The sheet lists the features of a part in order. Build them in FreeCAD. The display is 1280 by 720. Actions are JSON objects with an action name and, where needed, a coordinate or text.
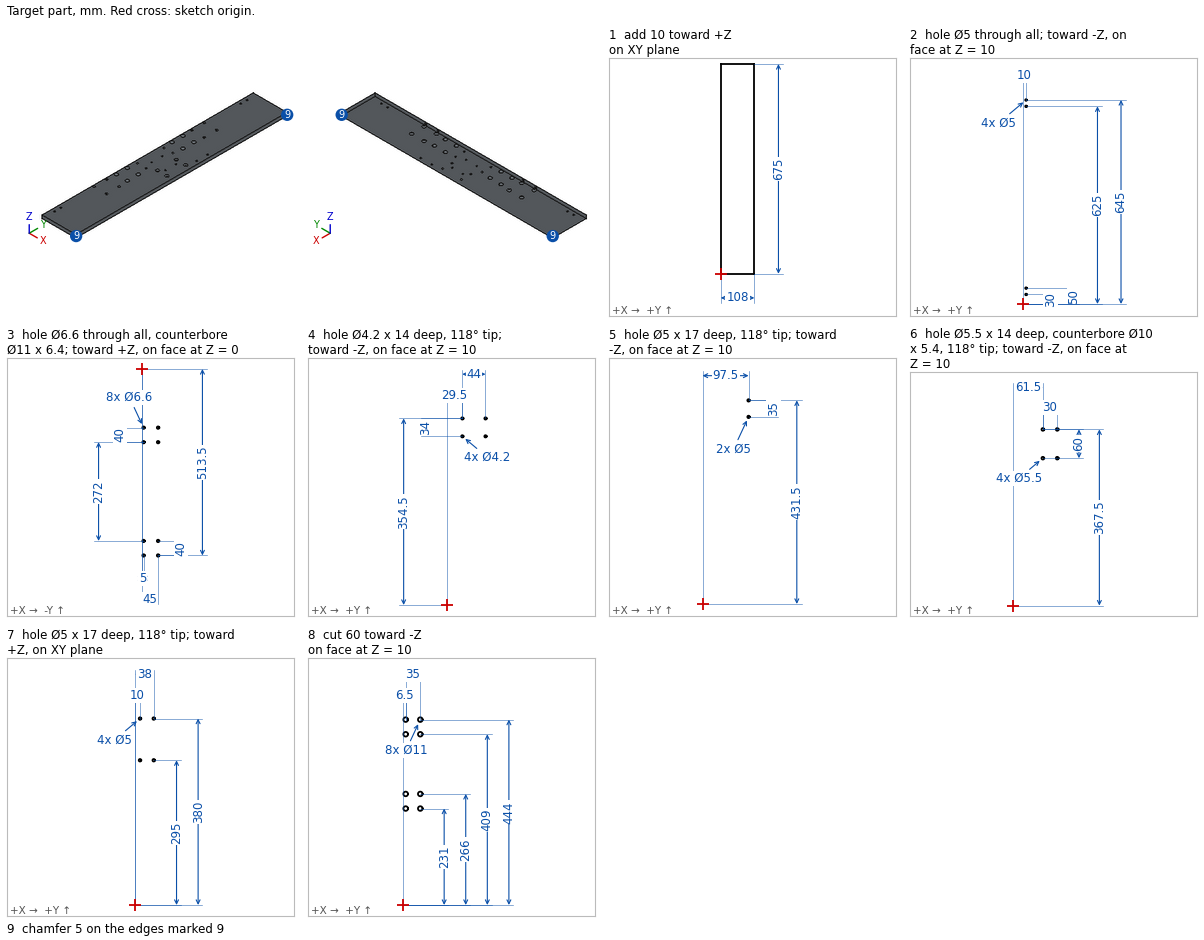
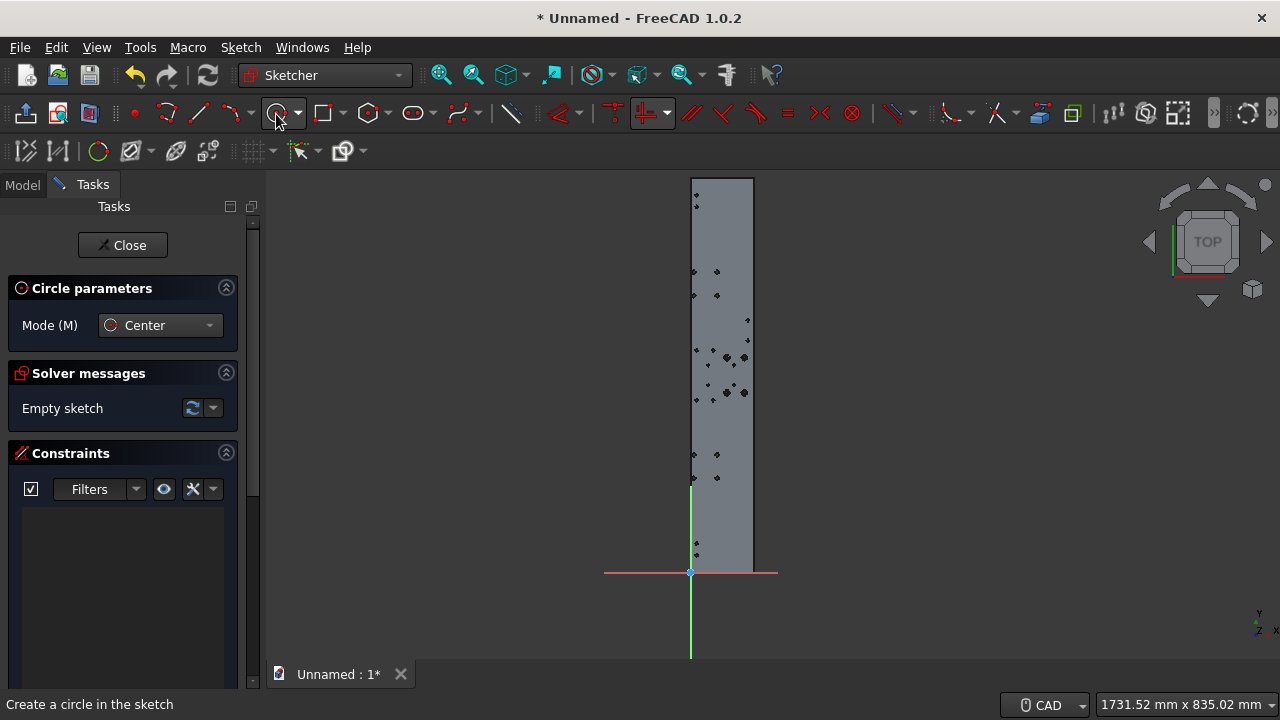
{"action": "scroll", "coordinate": [715, 313], "scroll_direction": "up", "scroll_amount": 10}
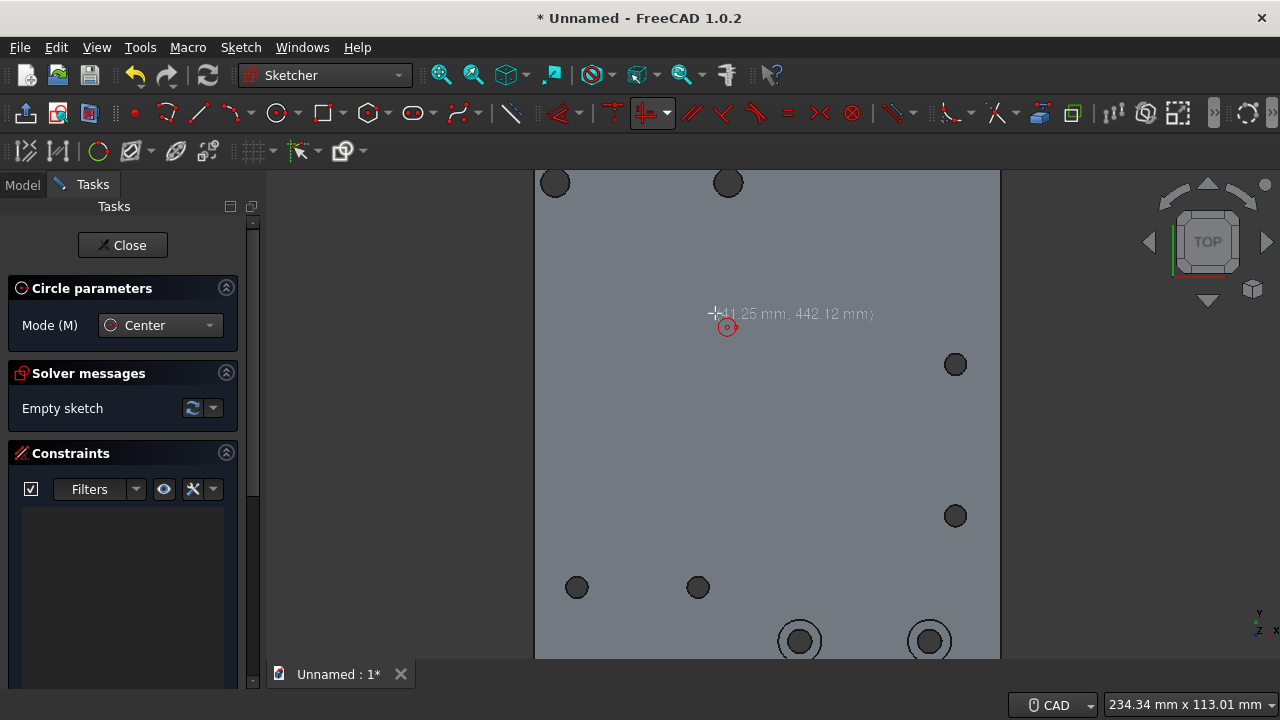
{"action": "scroll", "coordinate": [718, 247], "scroll_direction": "down", "scroll_amount": 9}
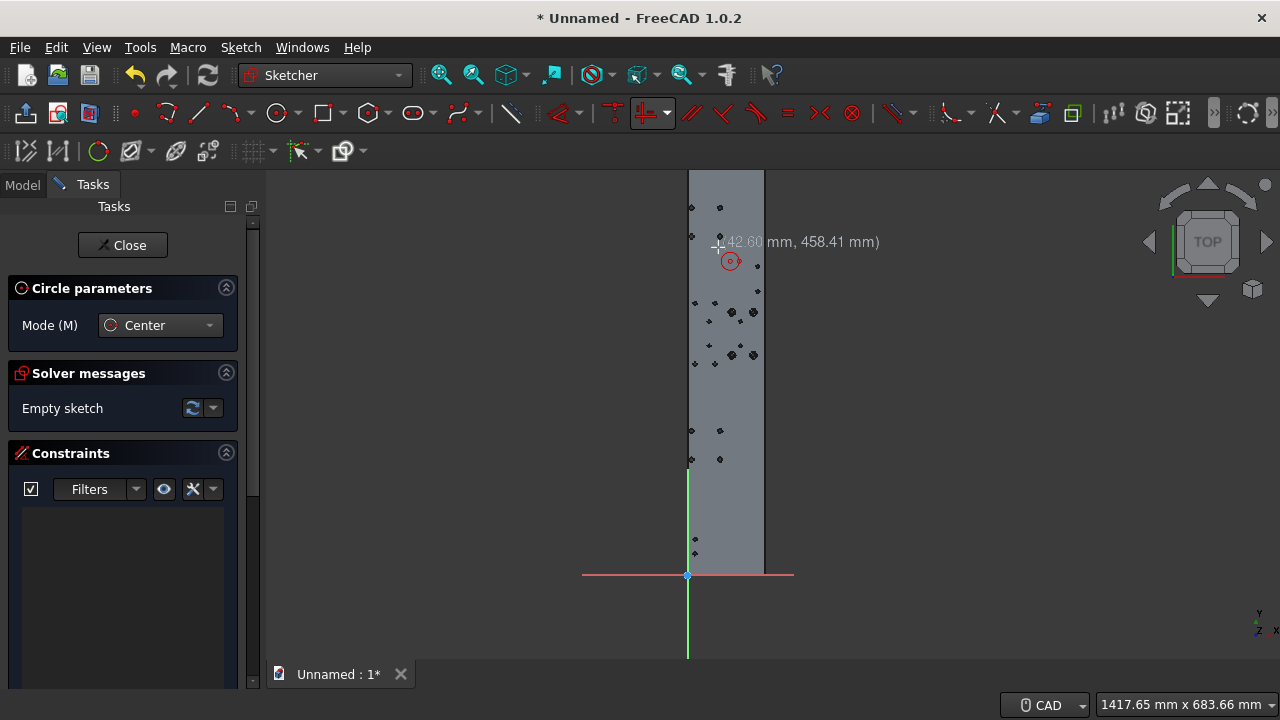
{"action": "left_click", "coordinate": [718, 258]}
{"action": "mouse_move", "coordinate": [720, 255]}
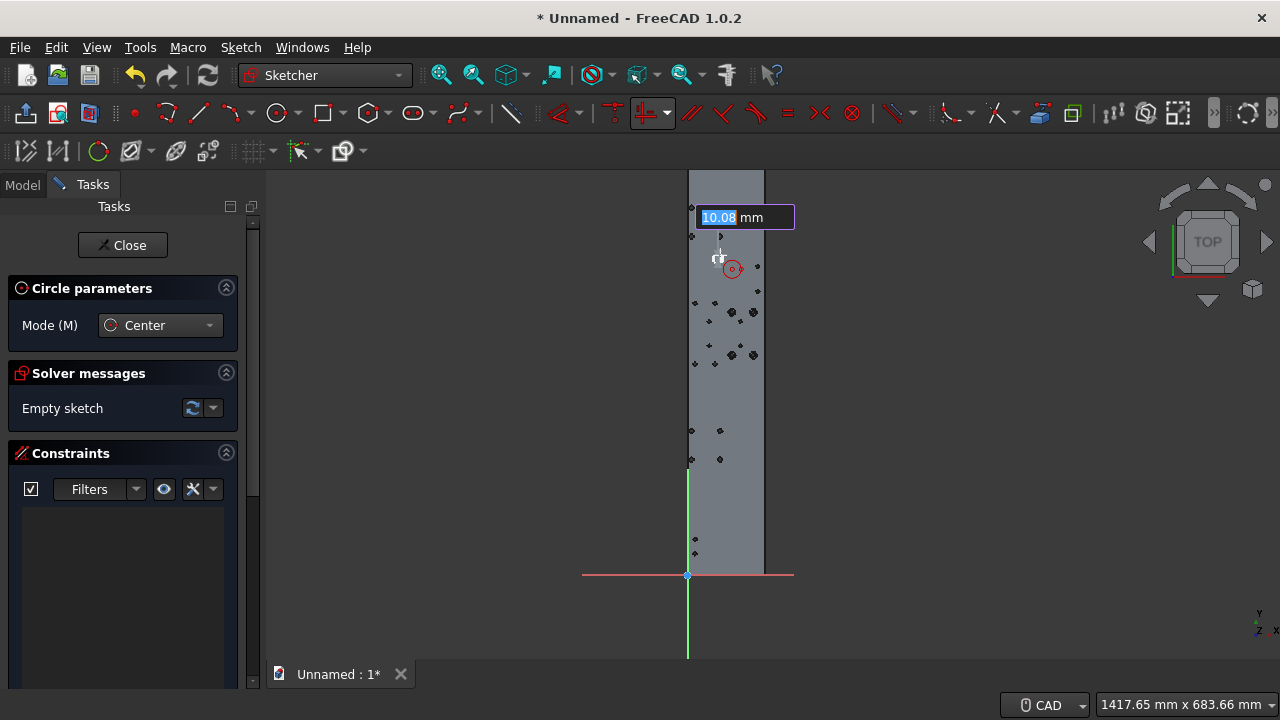
{"action": "type", "text": "11"}
{"action": "key", "text": "Return"}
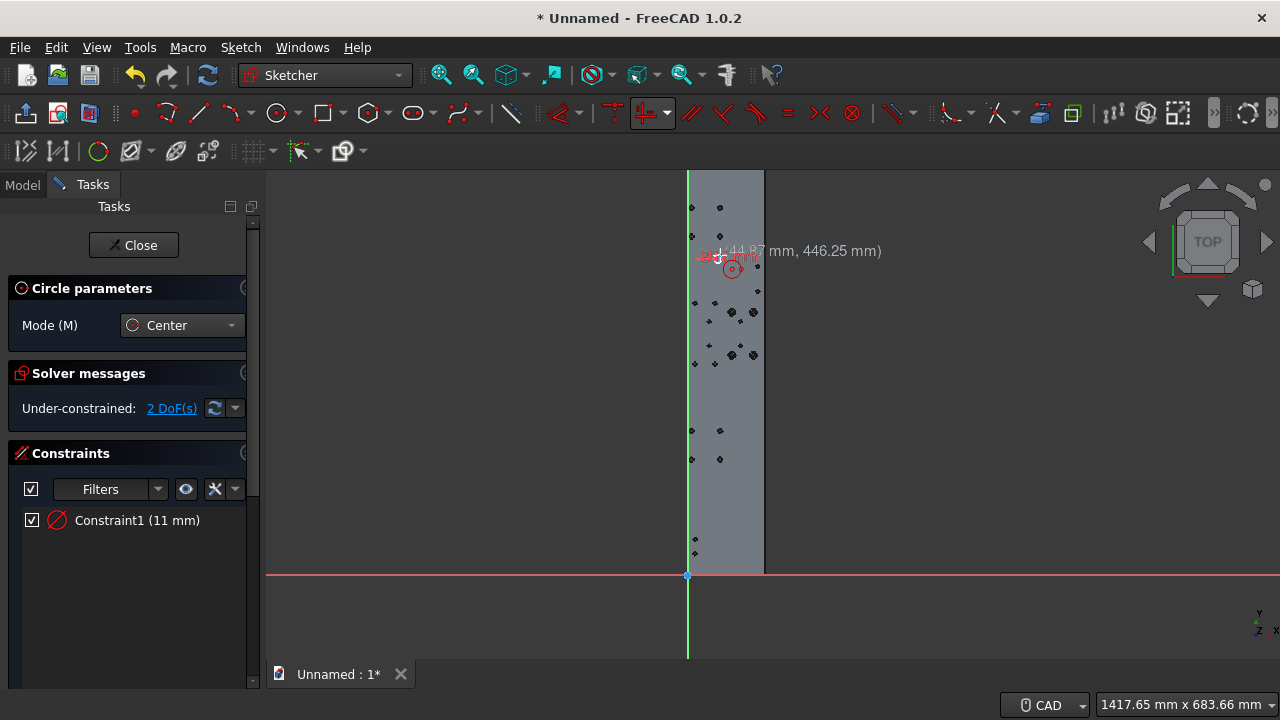
{"action": "scroll", "coordinate": [693, 258], "scroll_direction": "up", "scroll_amount": 9}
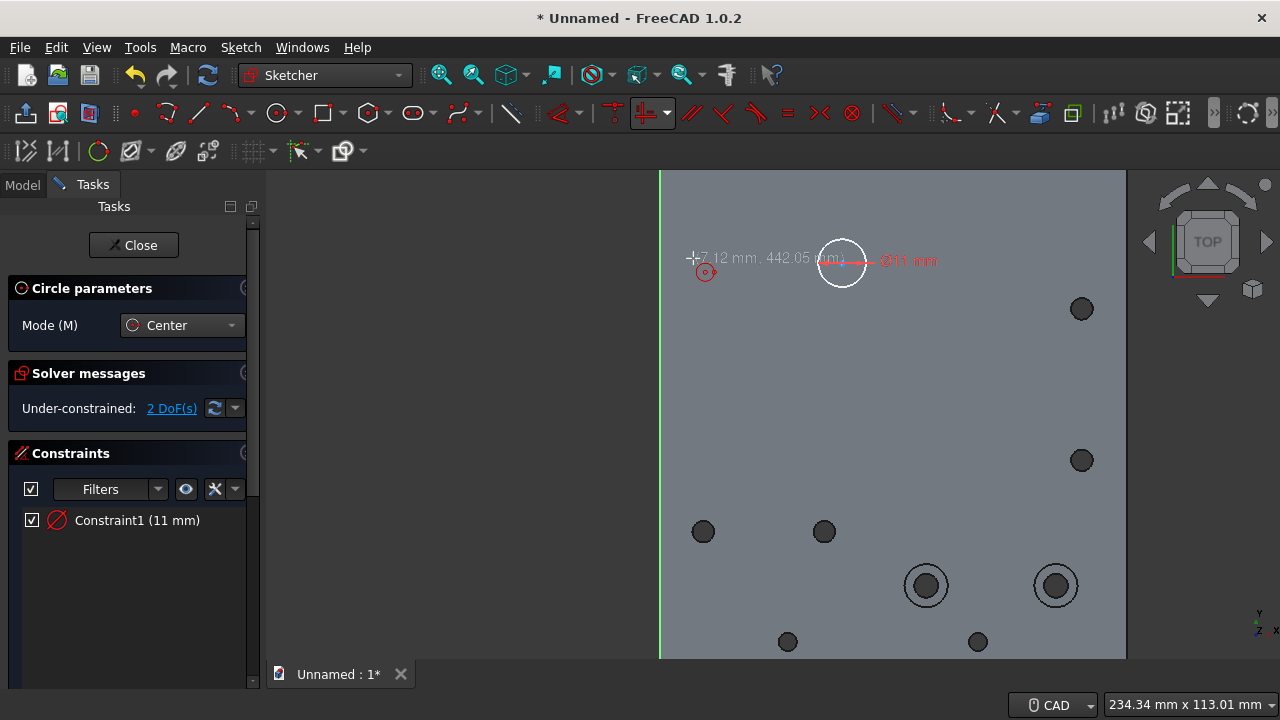
{"action": "left_click", "coordinate": [688, 255]}
{"action": "mouse_move", "coordinate": [705, 238]}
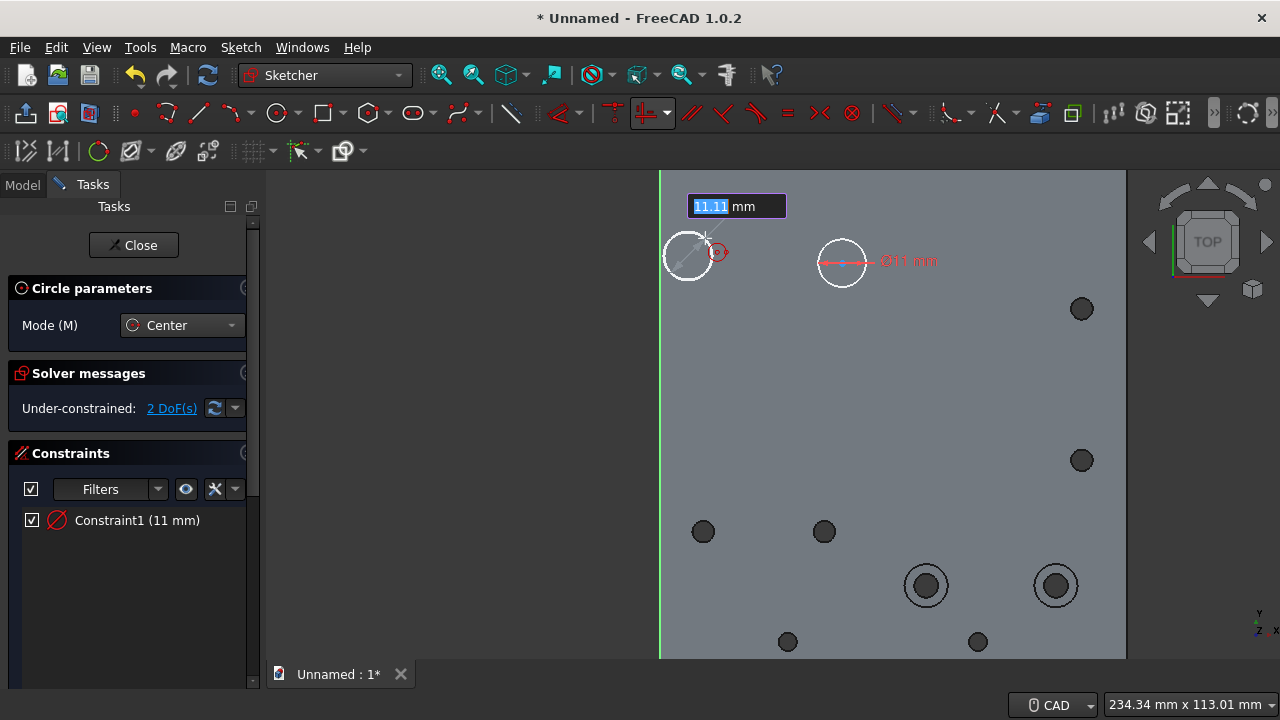
{"action": "type", "text": "11"}
{"action": "key", "text": "Return"}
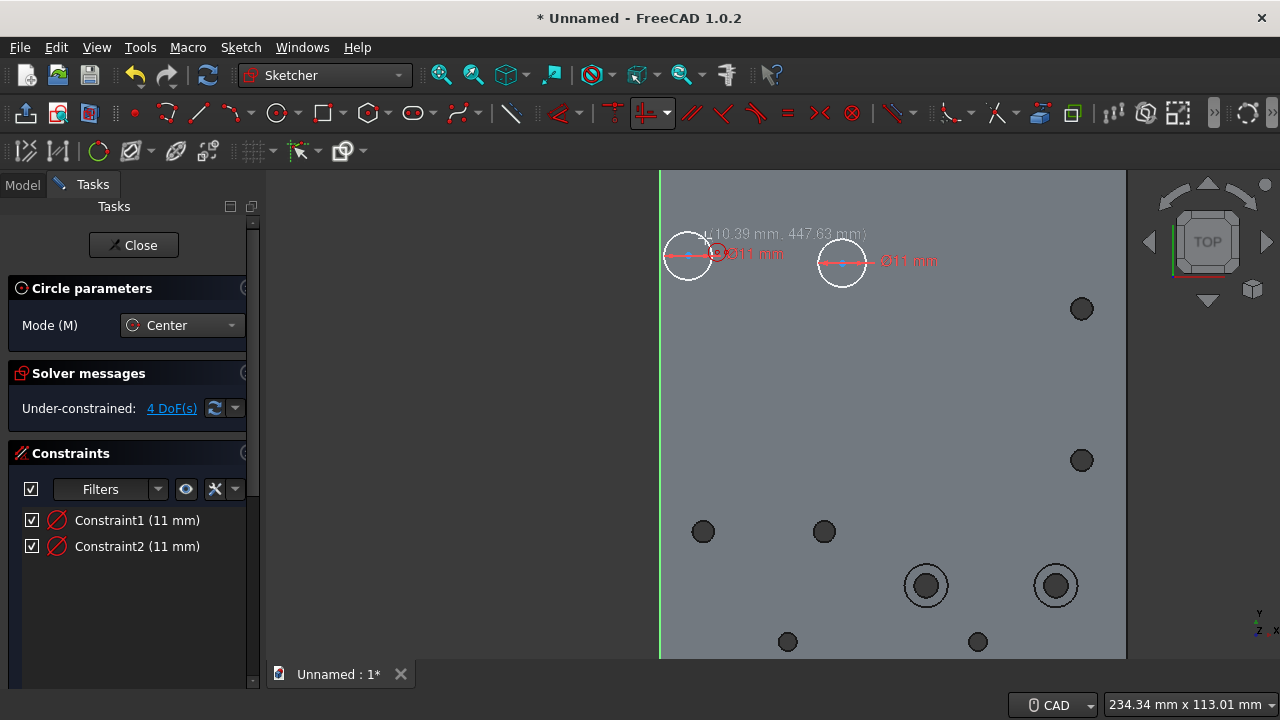
{"action": "scroll", "coordinate": [693, 258], "scroll_direction": "down", "scroll_amount": 9}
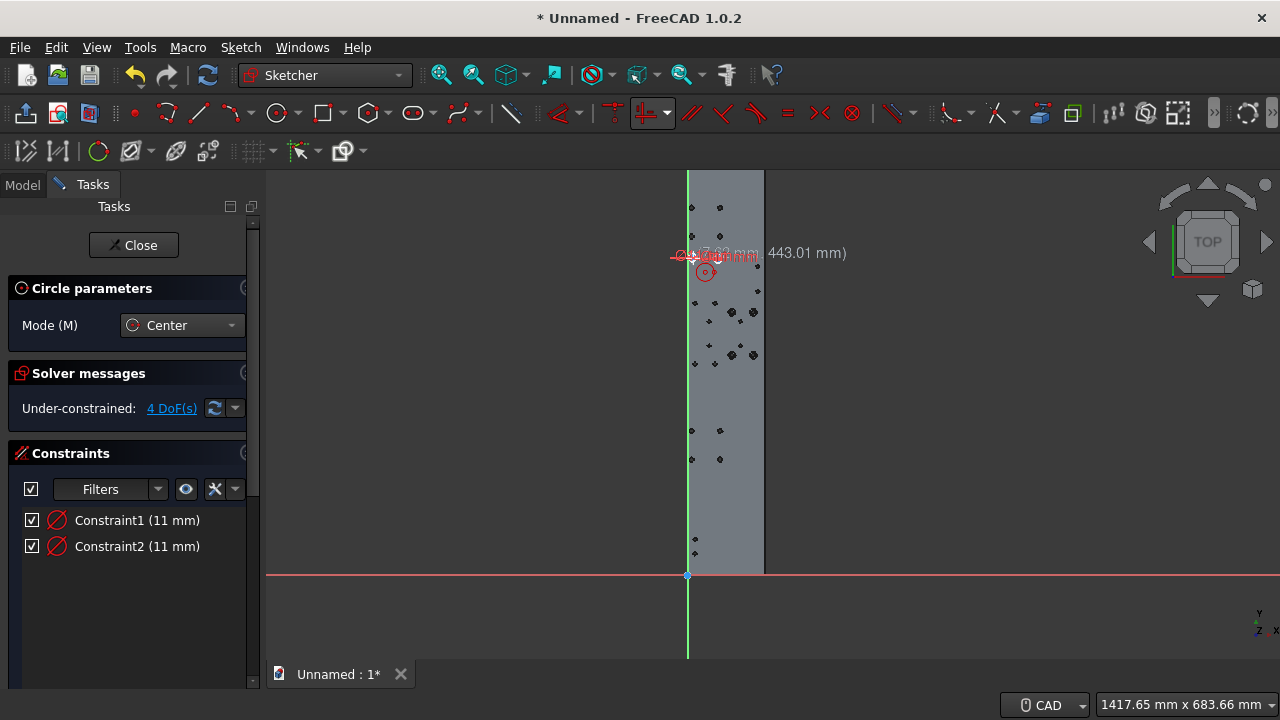
{"action": "left_click", "coordinate": [718, 283]}
{"action": "mouse_move", "coordinate": [720, 280]}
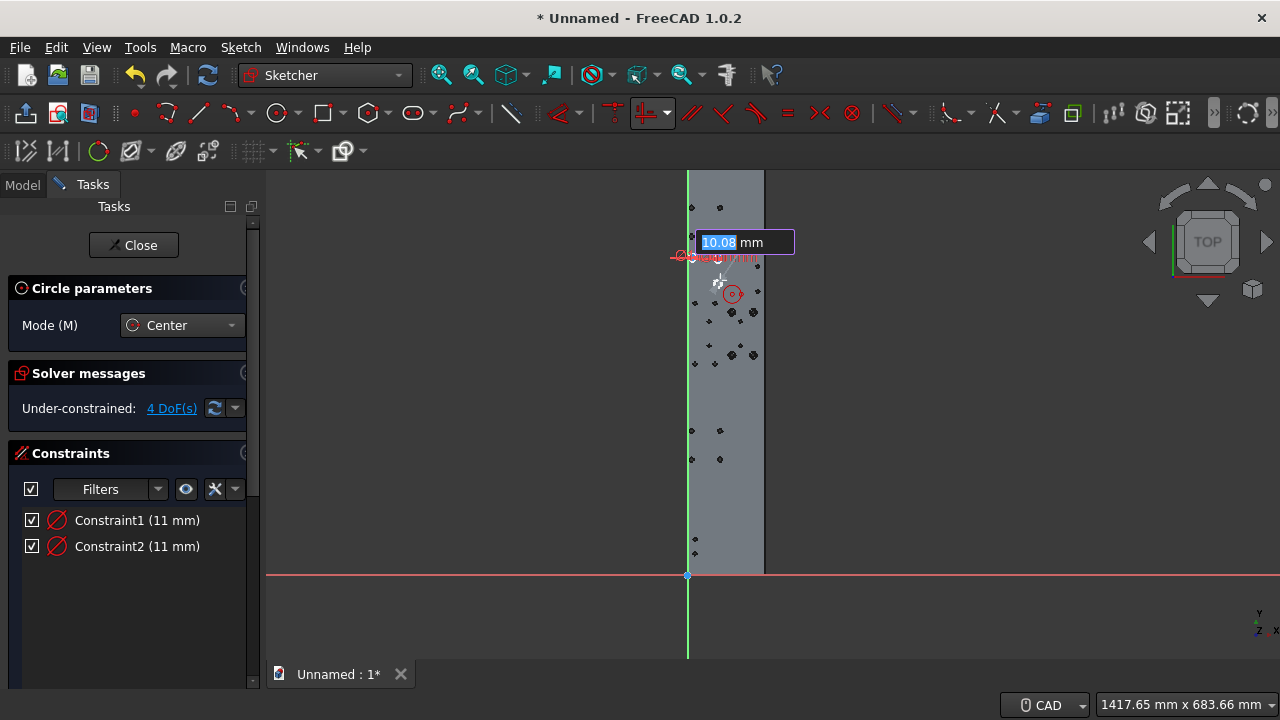
{"action": "type", "text": "11"}
{"action": "key", "text": "Return"}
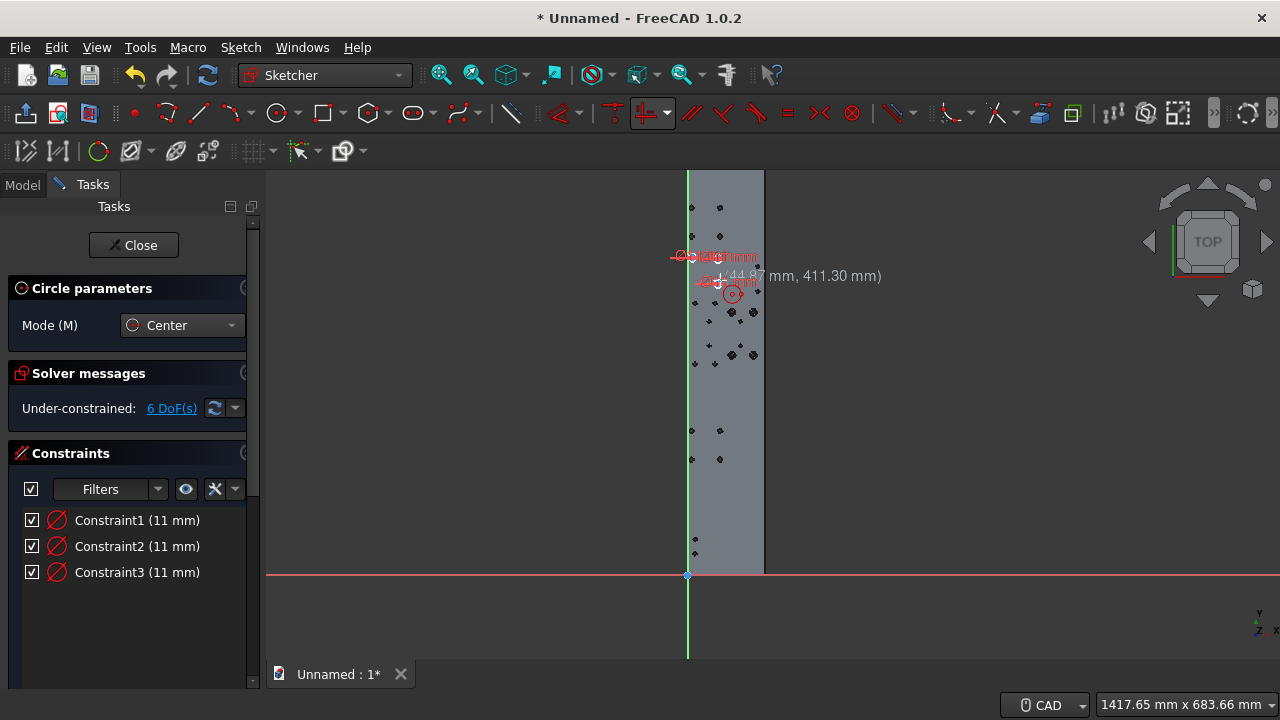
{"action": "scroll", "coordinate": [693, 283], "scroll_direction": "up", "scroll_amount": 9}